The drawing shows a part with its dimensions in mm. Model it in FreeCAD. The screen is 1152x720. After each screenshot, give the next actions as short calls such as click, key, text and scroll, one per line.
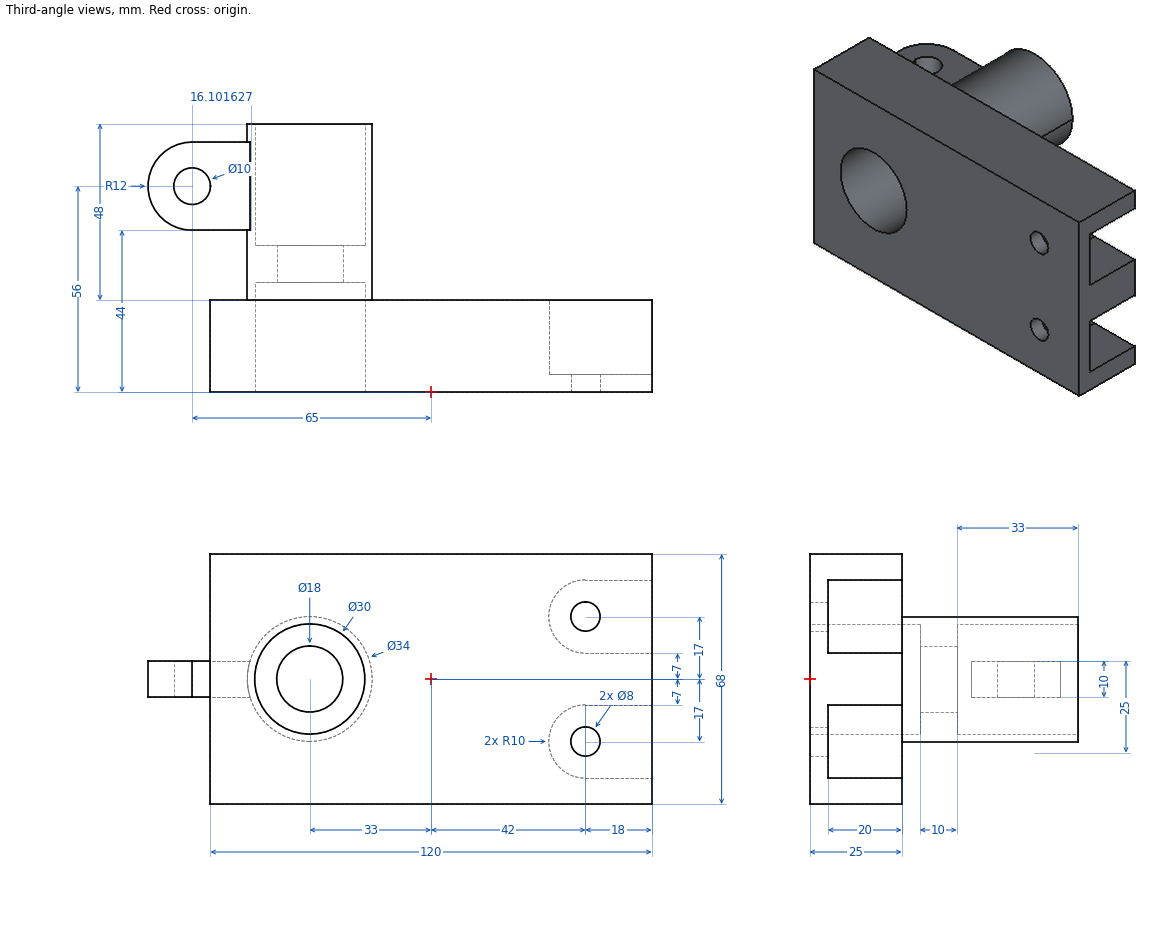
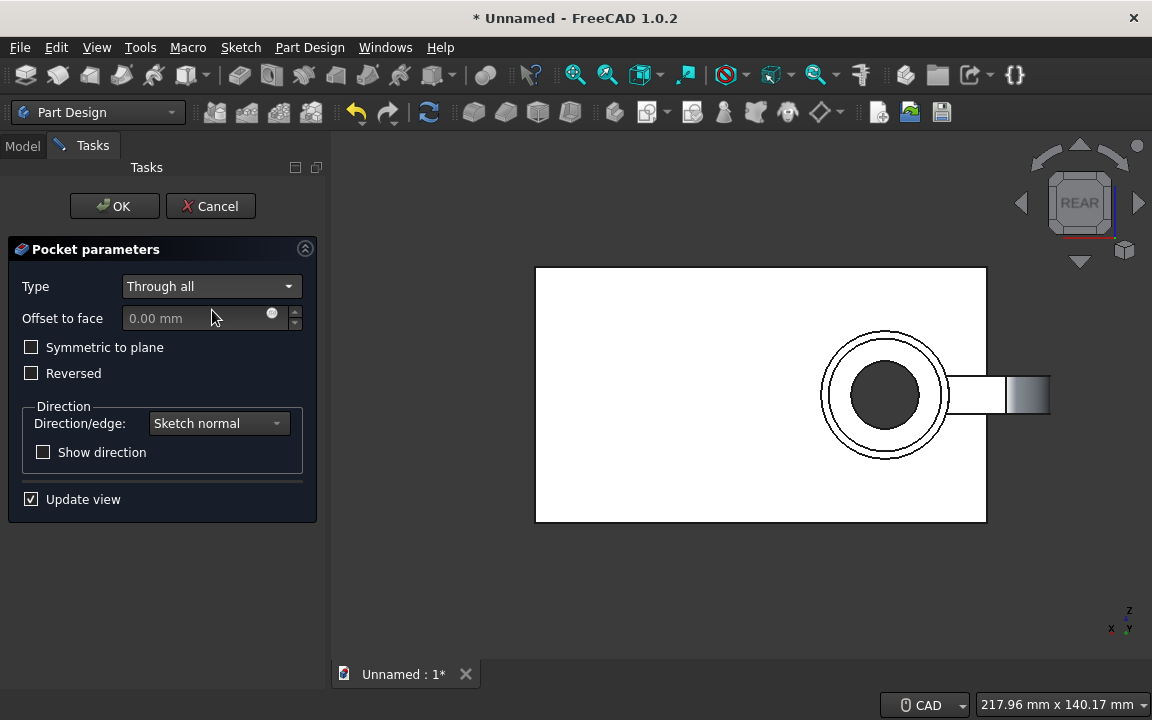
click(115, 206)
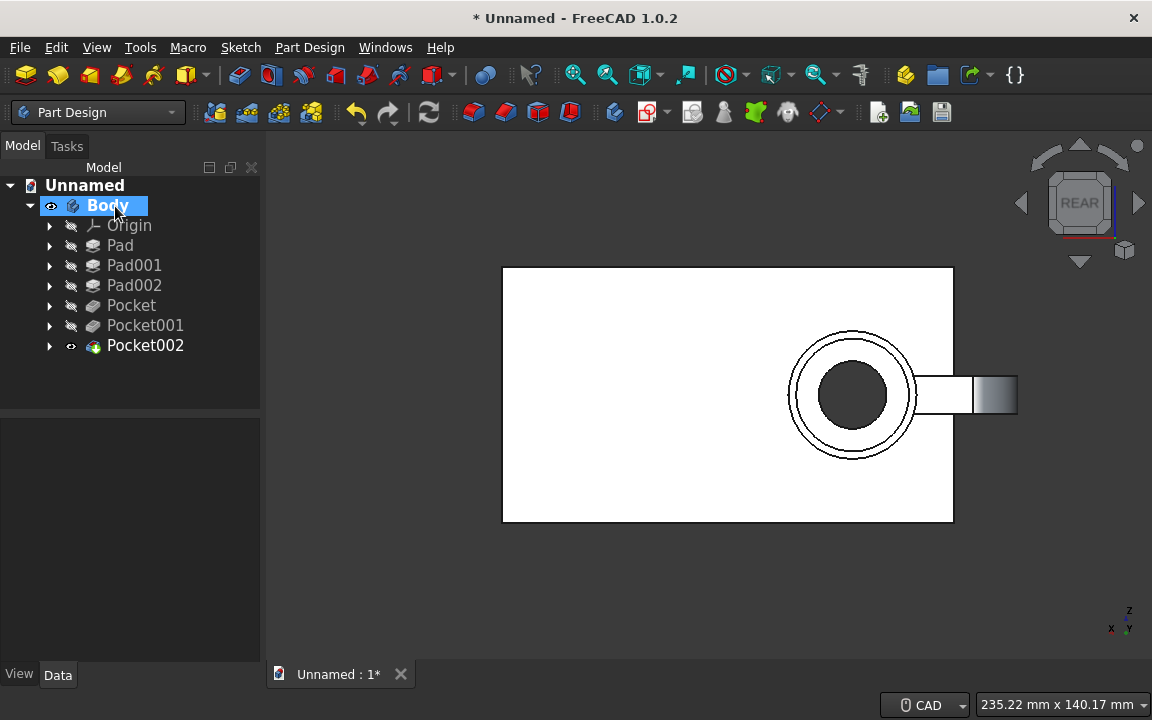
key(0)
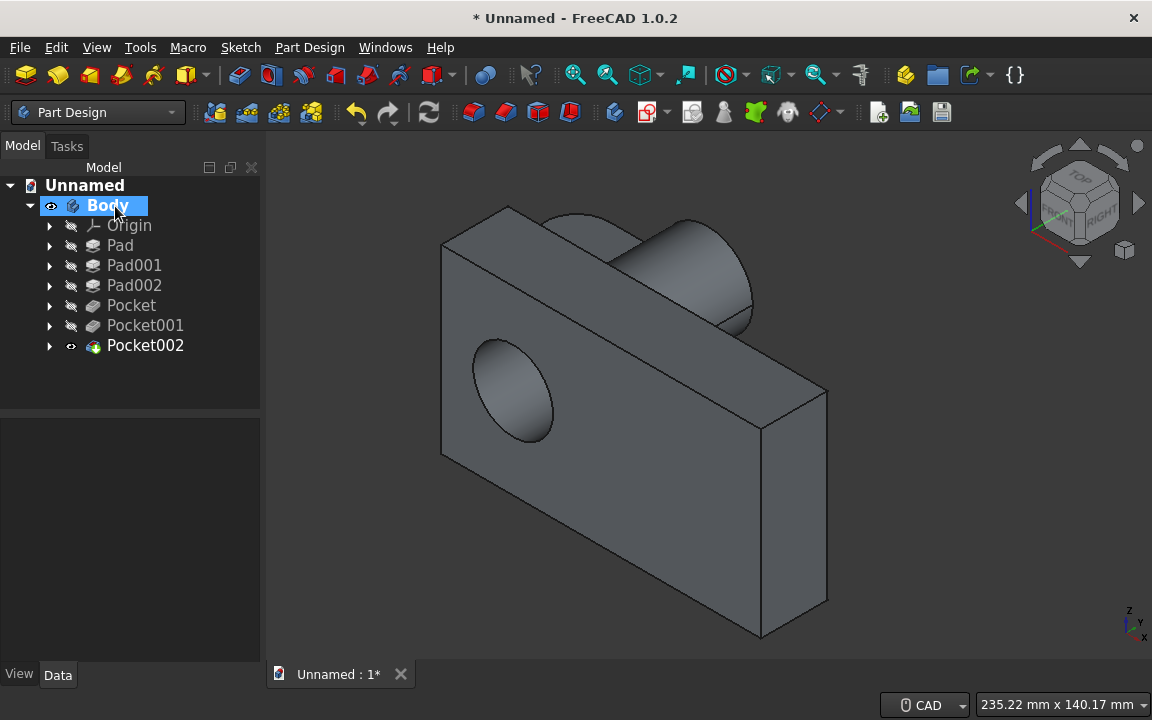
click(576, 76)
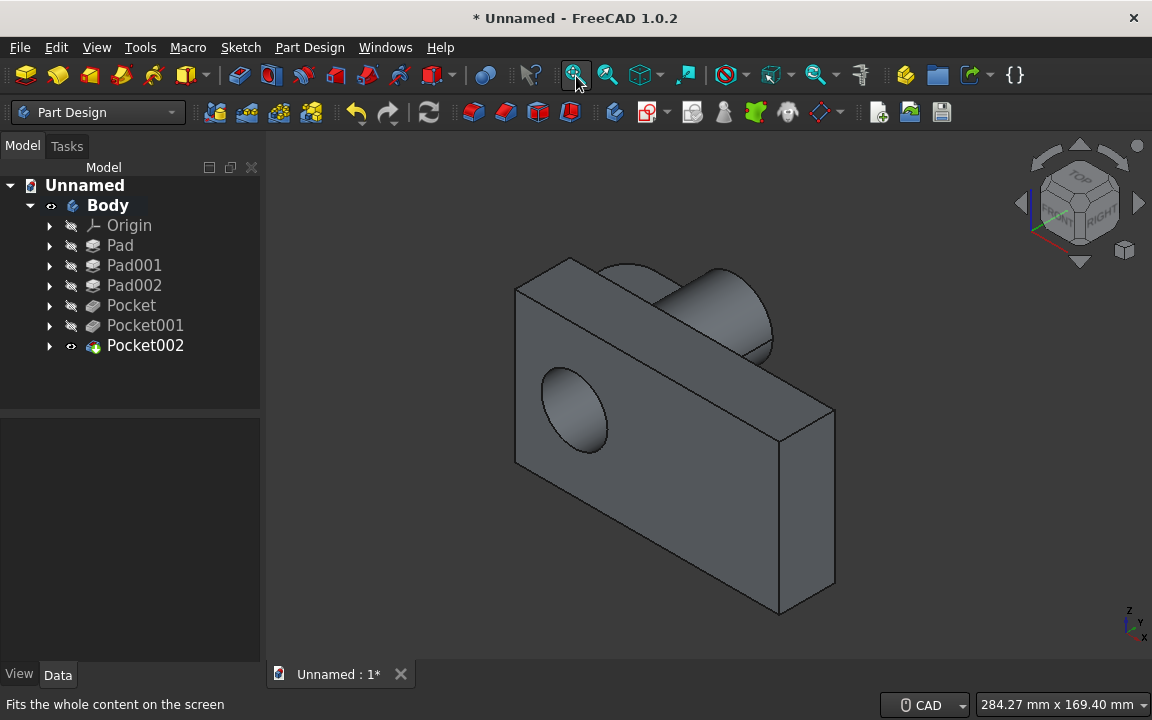
click(648, 288)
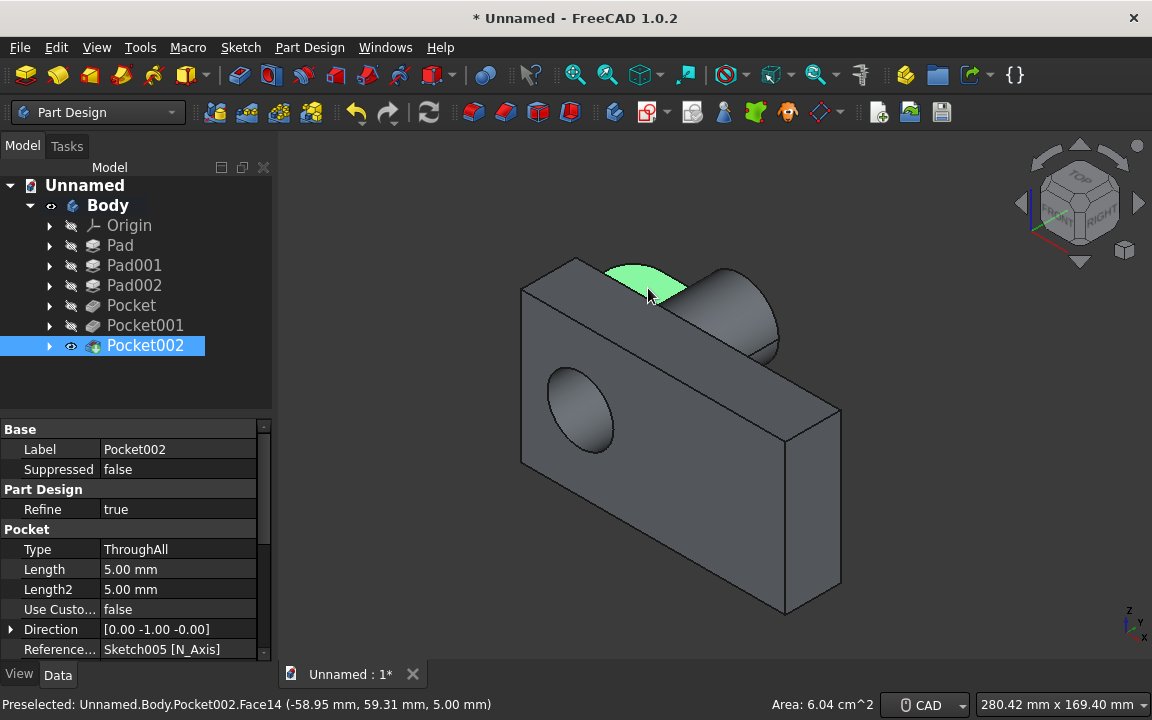
click(648, 112)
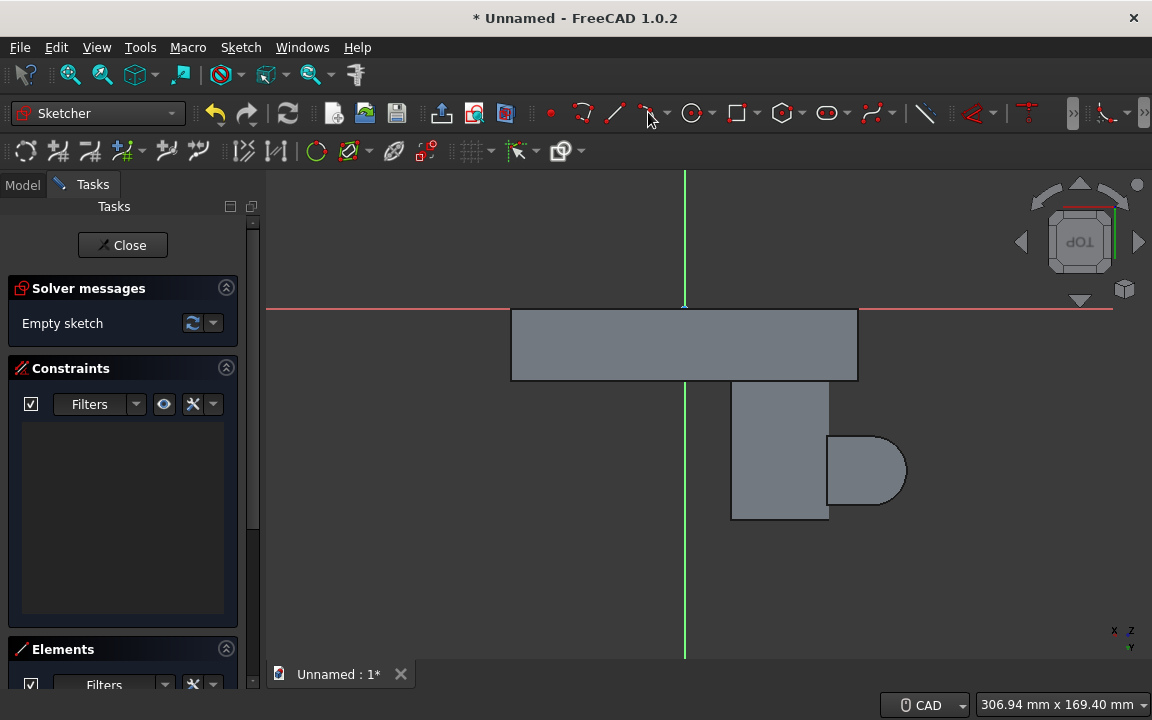
click(506, 114)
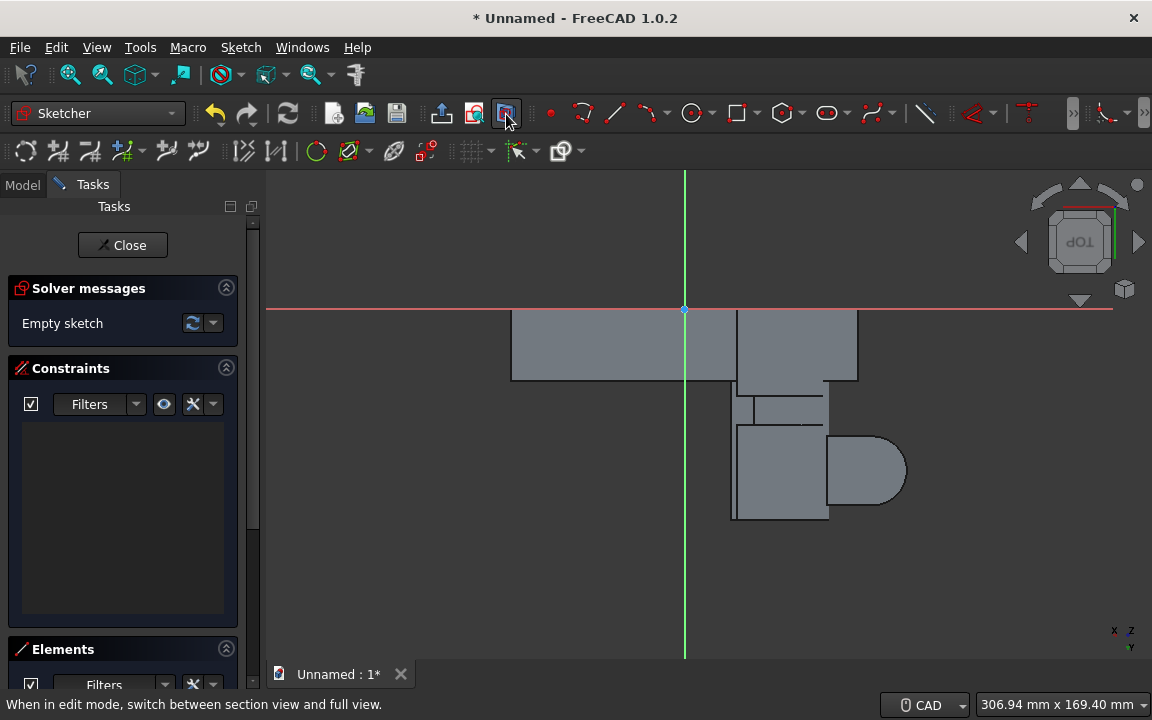
scroll(895, 476, up, 12)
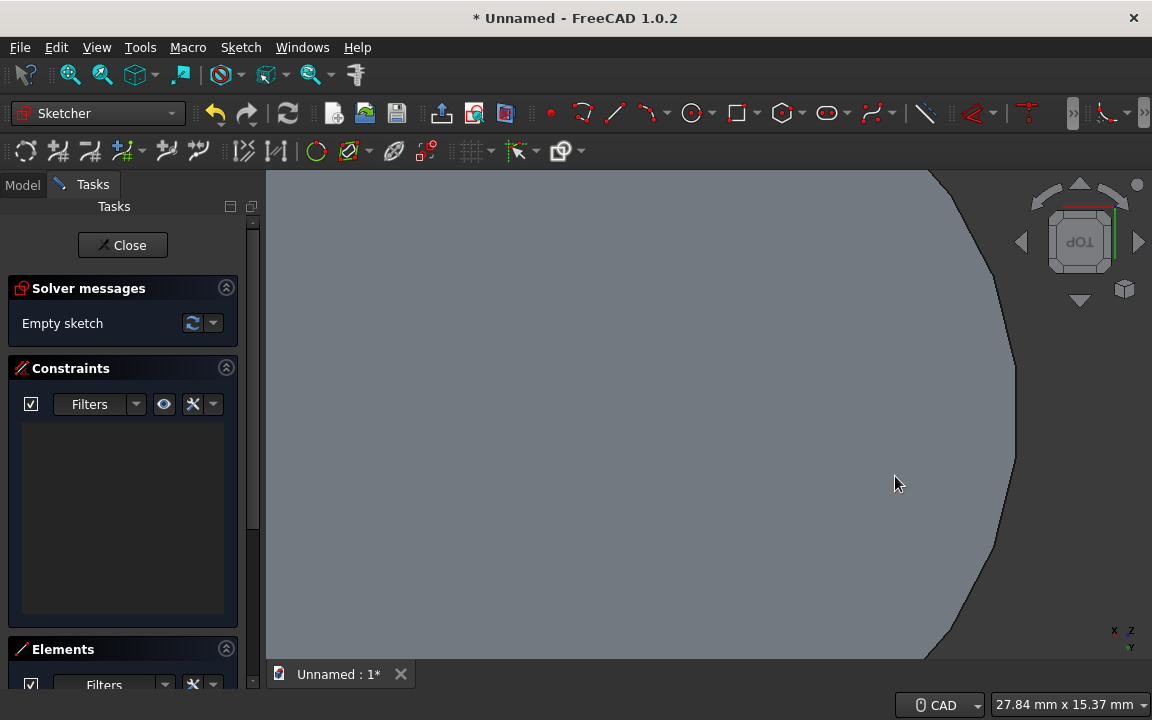
click(692, 114)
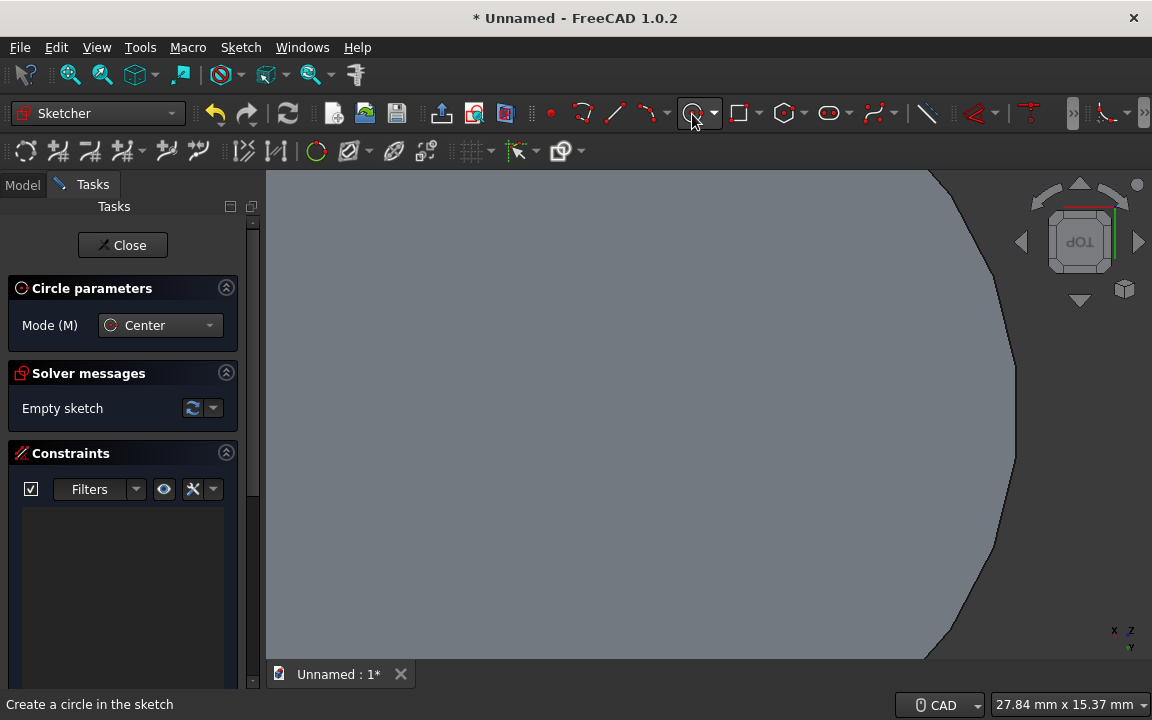
click(637, 412)
move(749, 300)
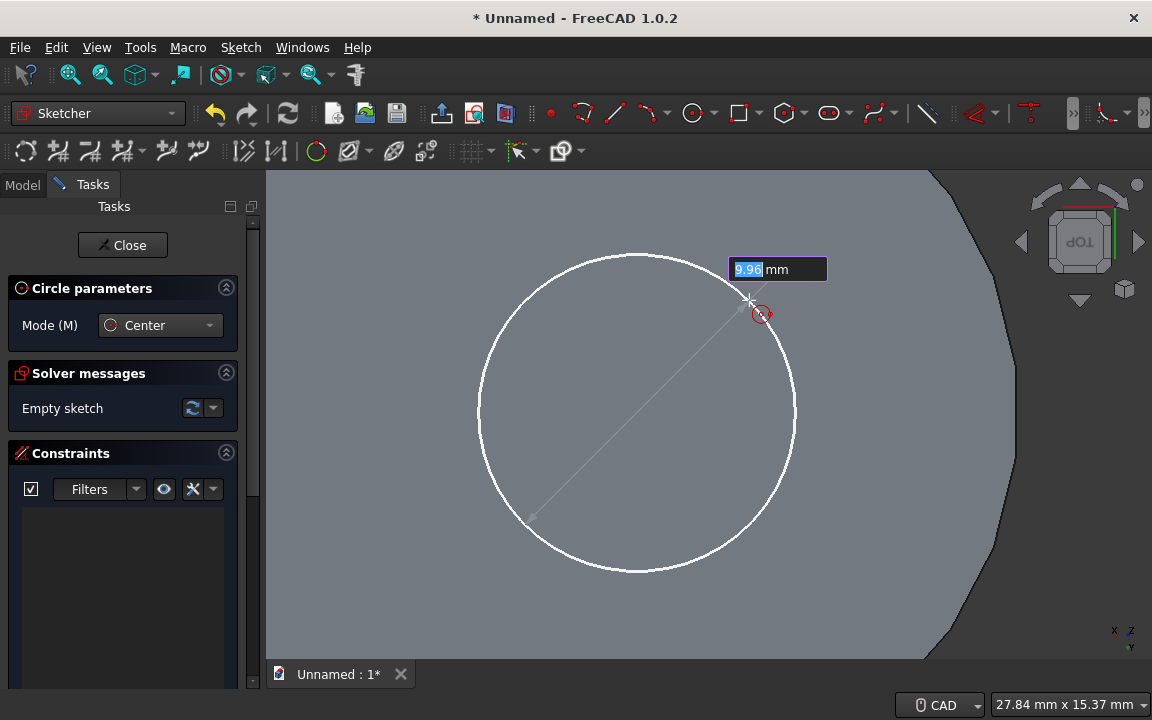
text(10)
key(Return)
key(Escape)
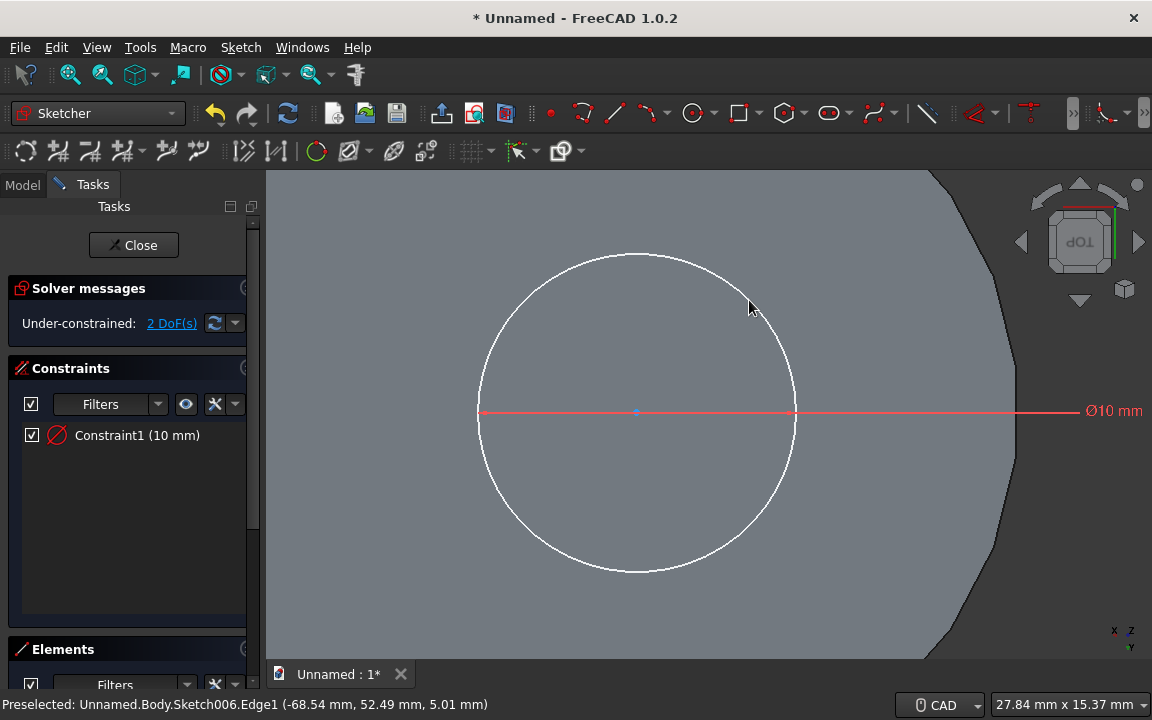
click(974, 114)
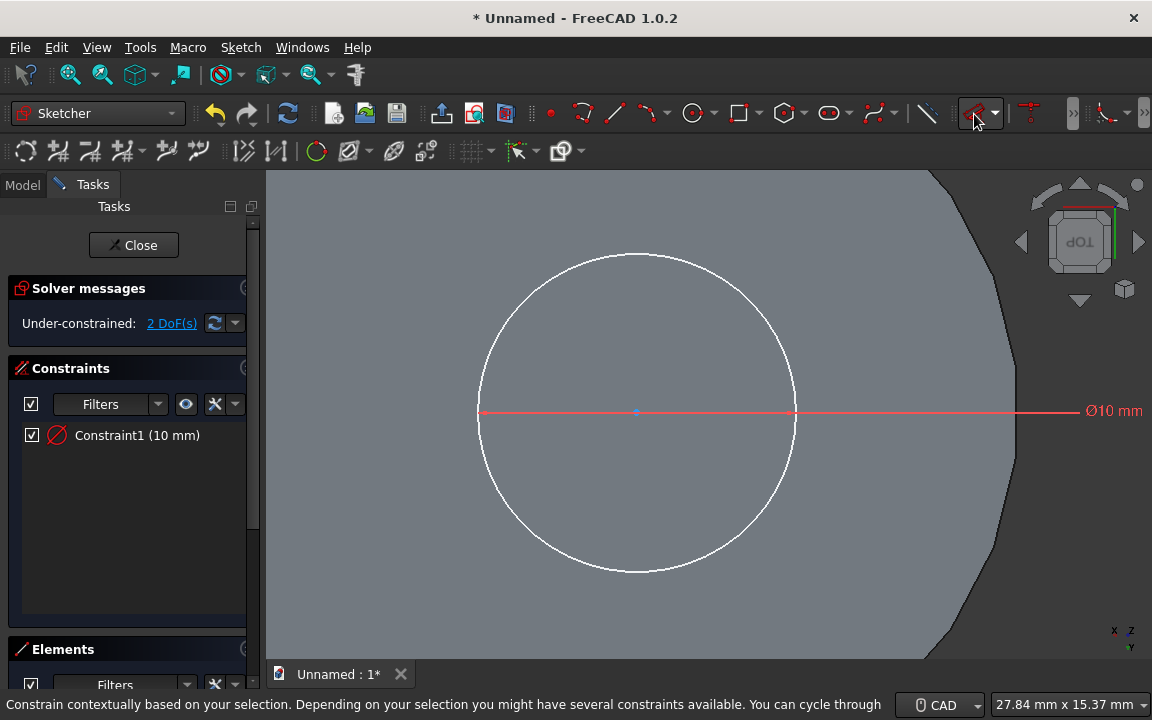
click(637, 413)
click(465, 447)